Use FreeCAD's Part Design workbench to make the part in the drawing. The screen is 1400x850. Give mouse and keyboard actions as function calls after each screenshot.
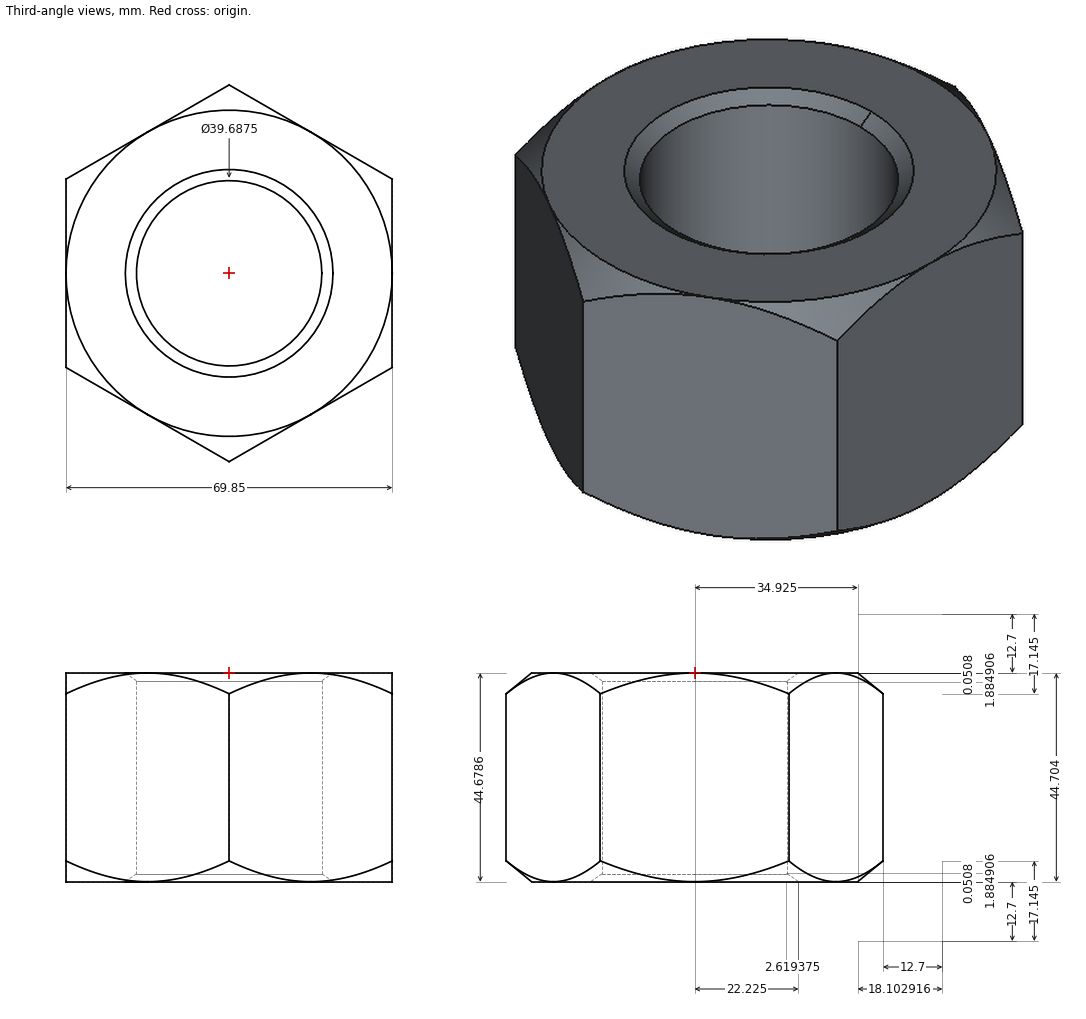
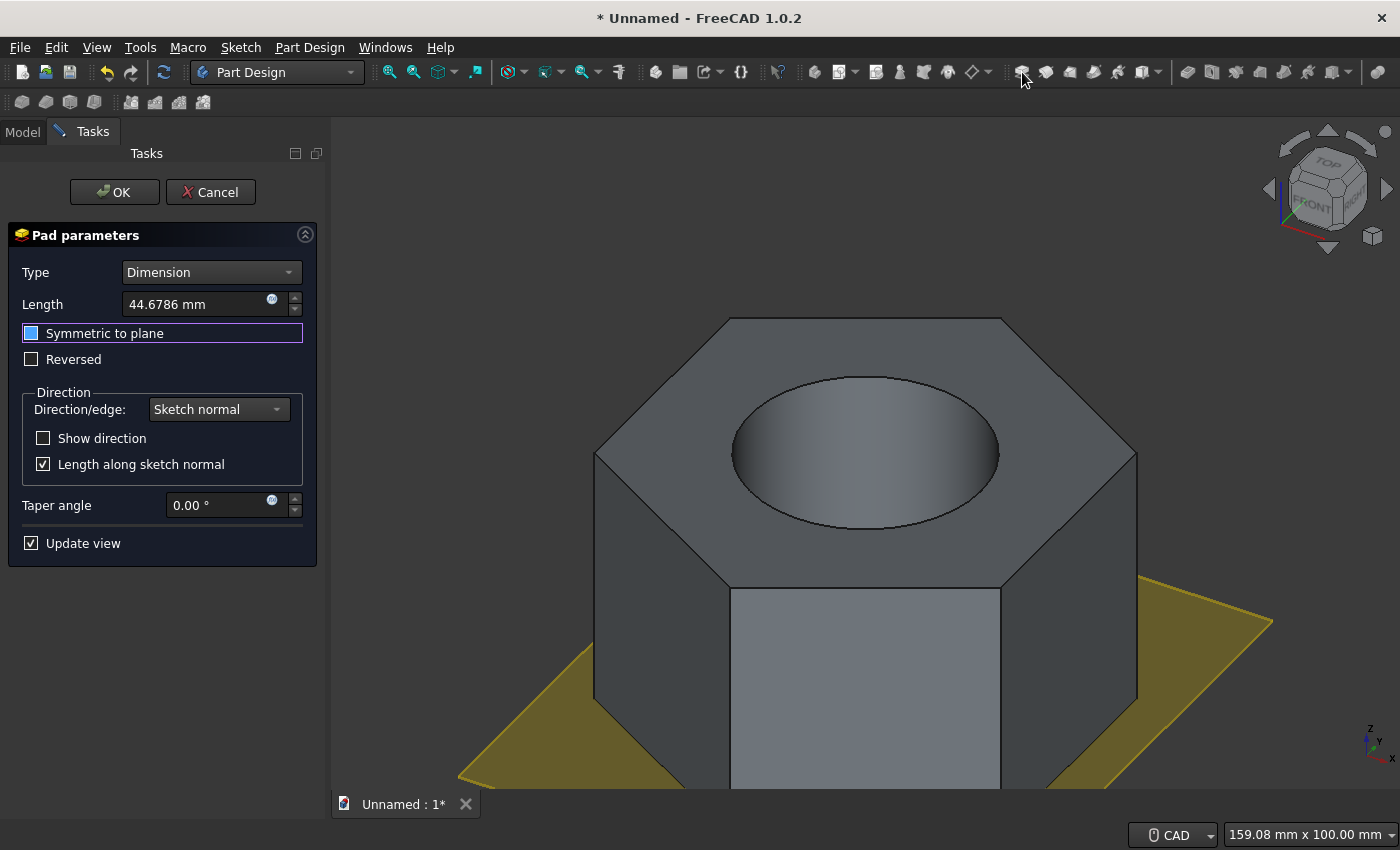
click(115, 192)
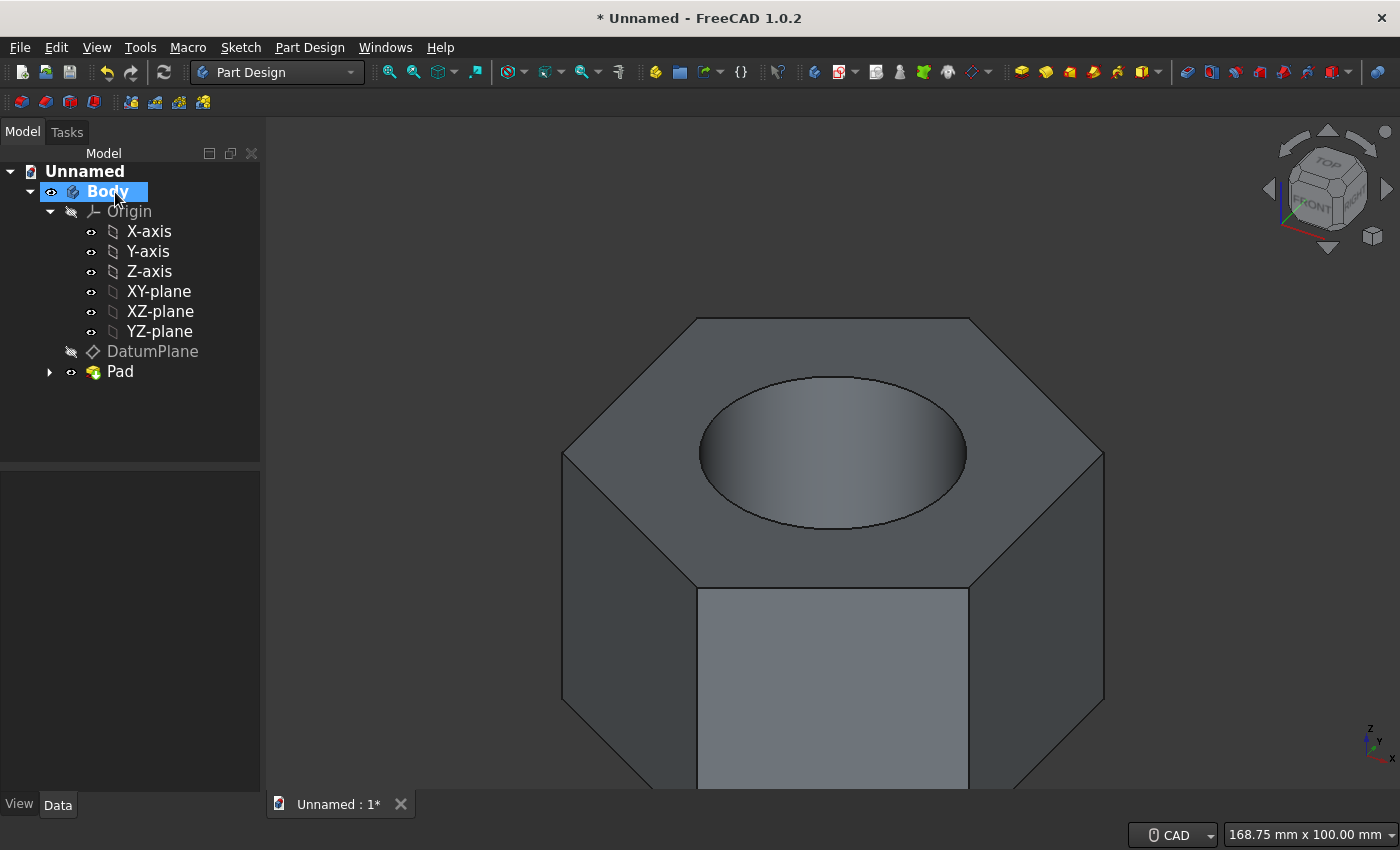
click(390, 72)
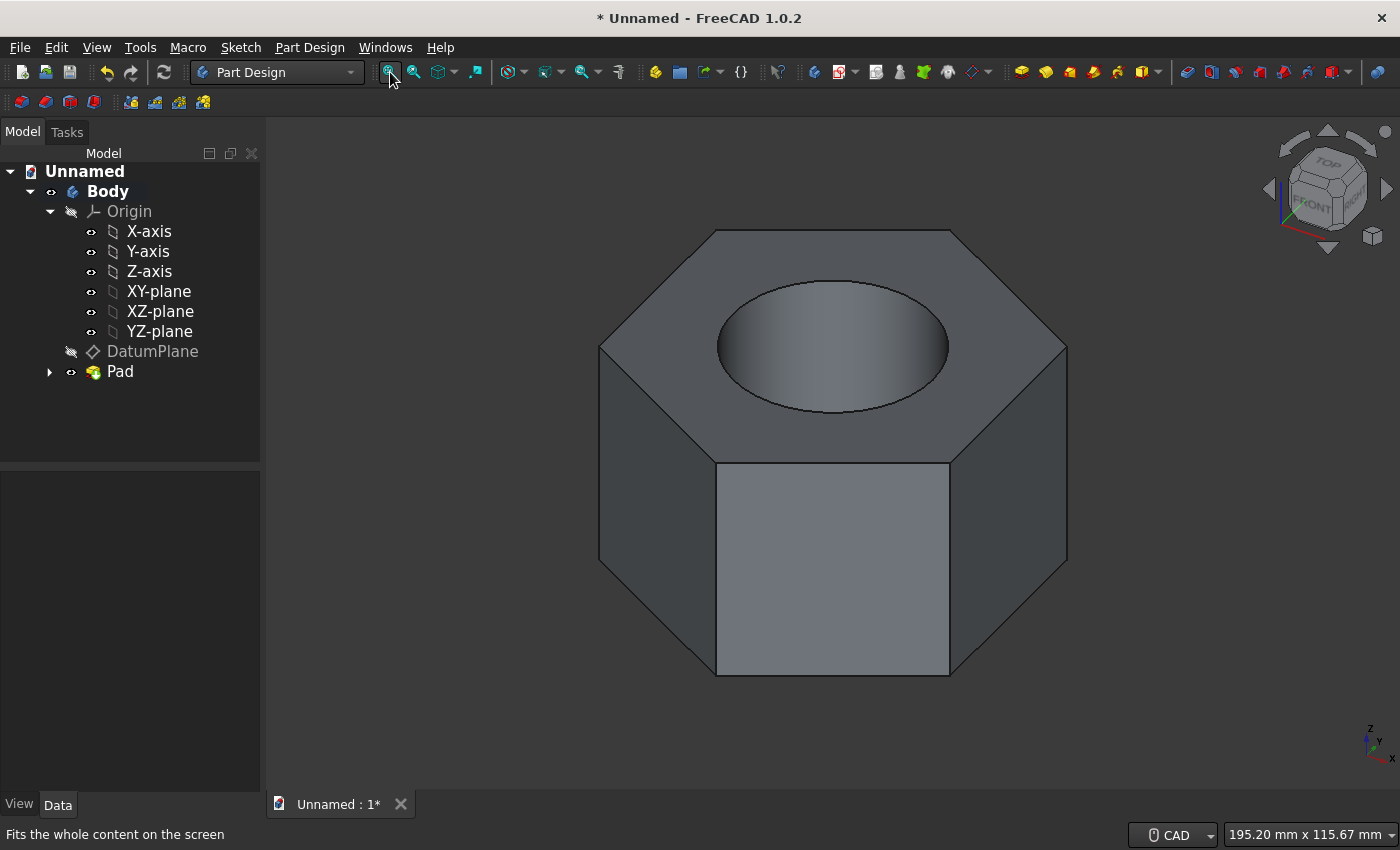
click(840, 72)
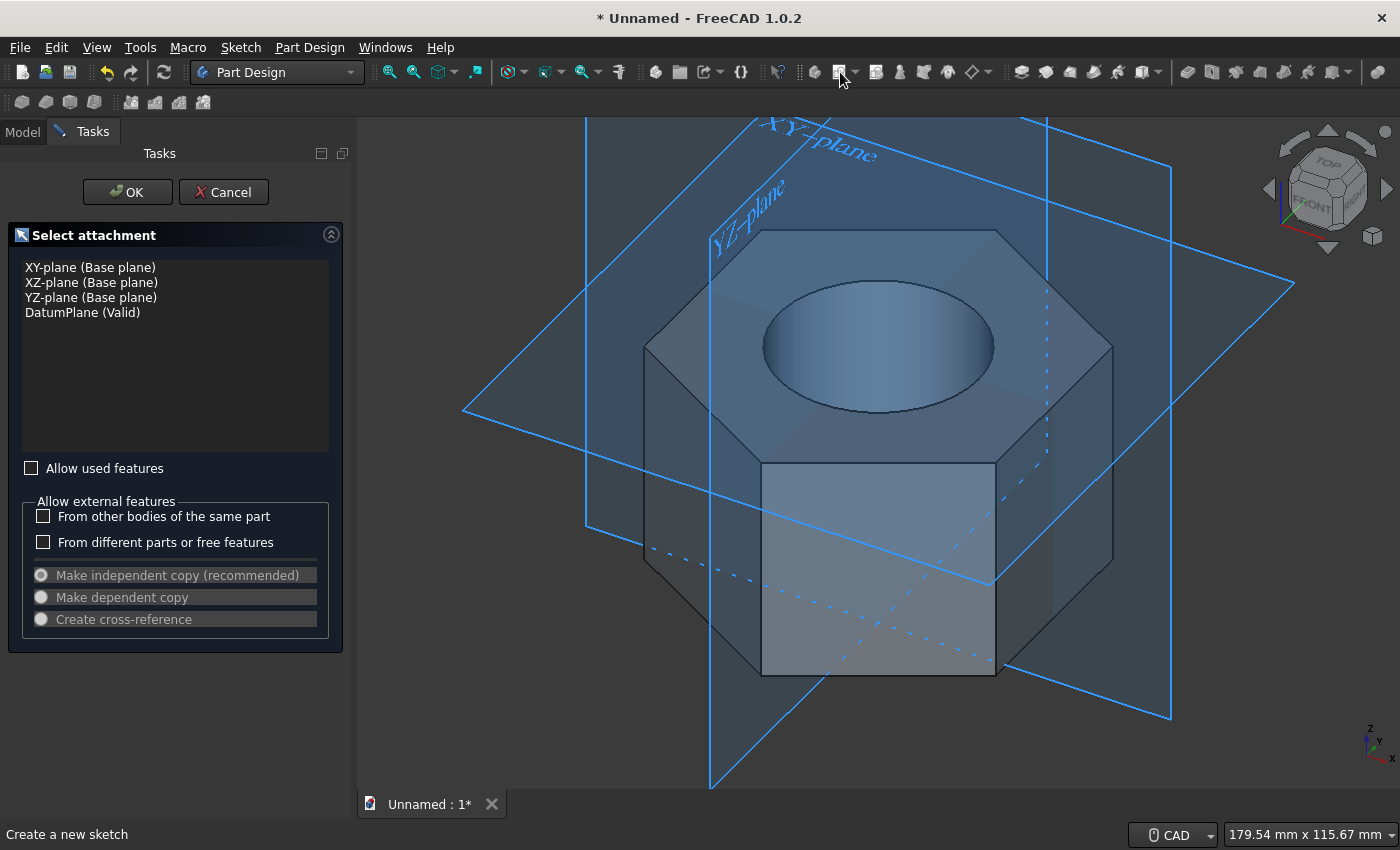
click(82, 298)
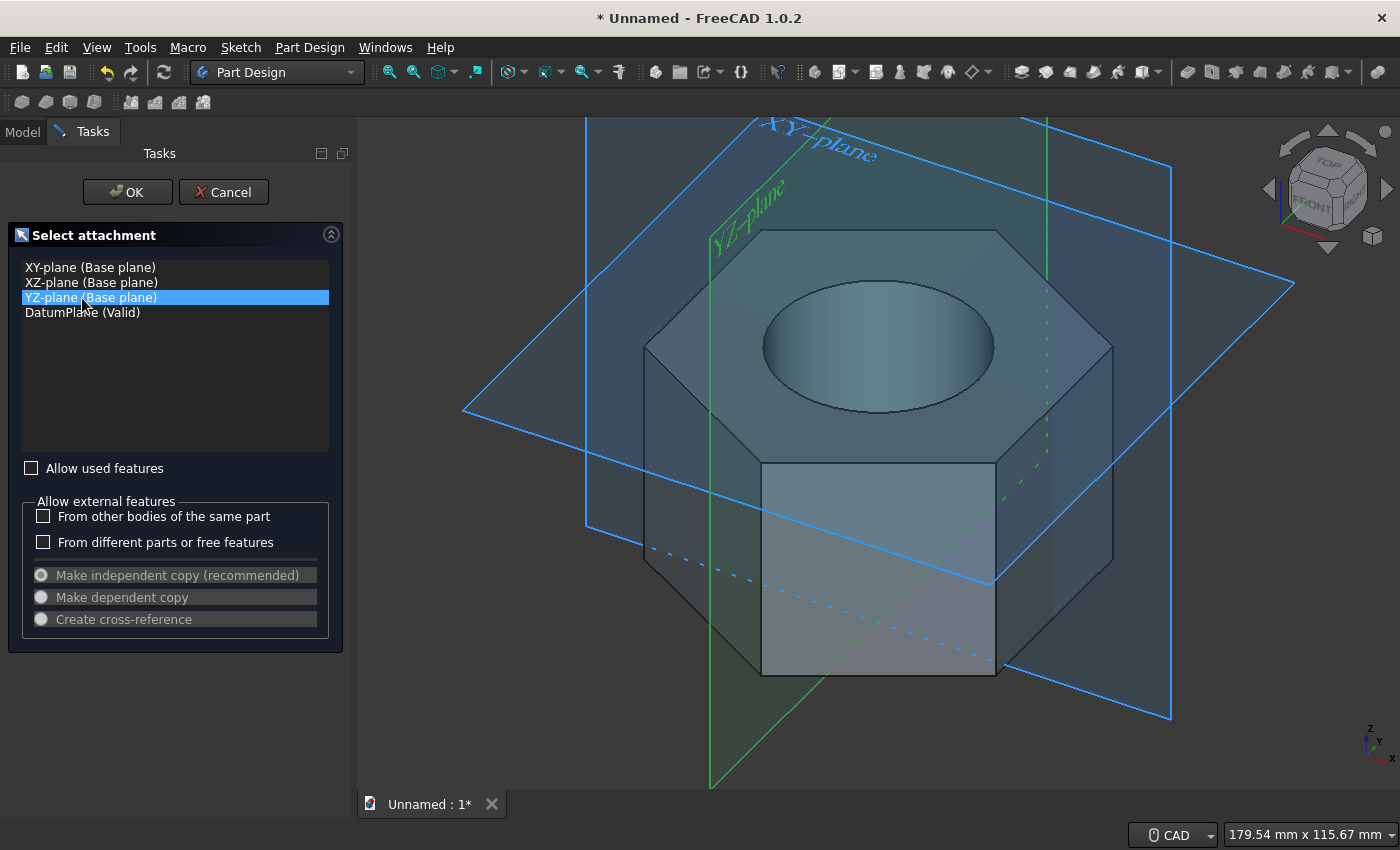
click(128, 192)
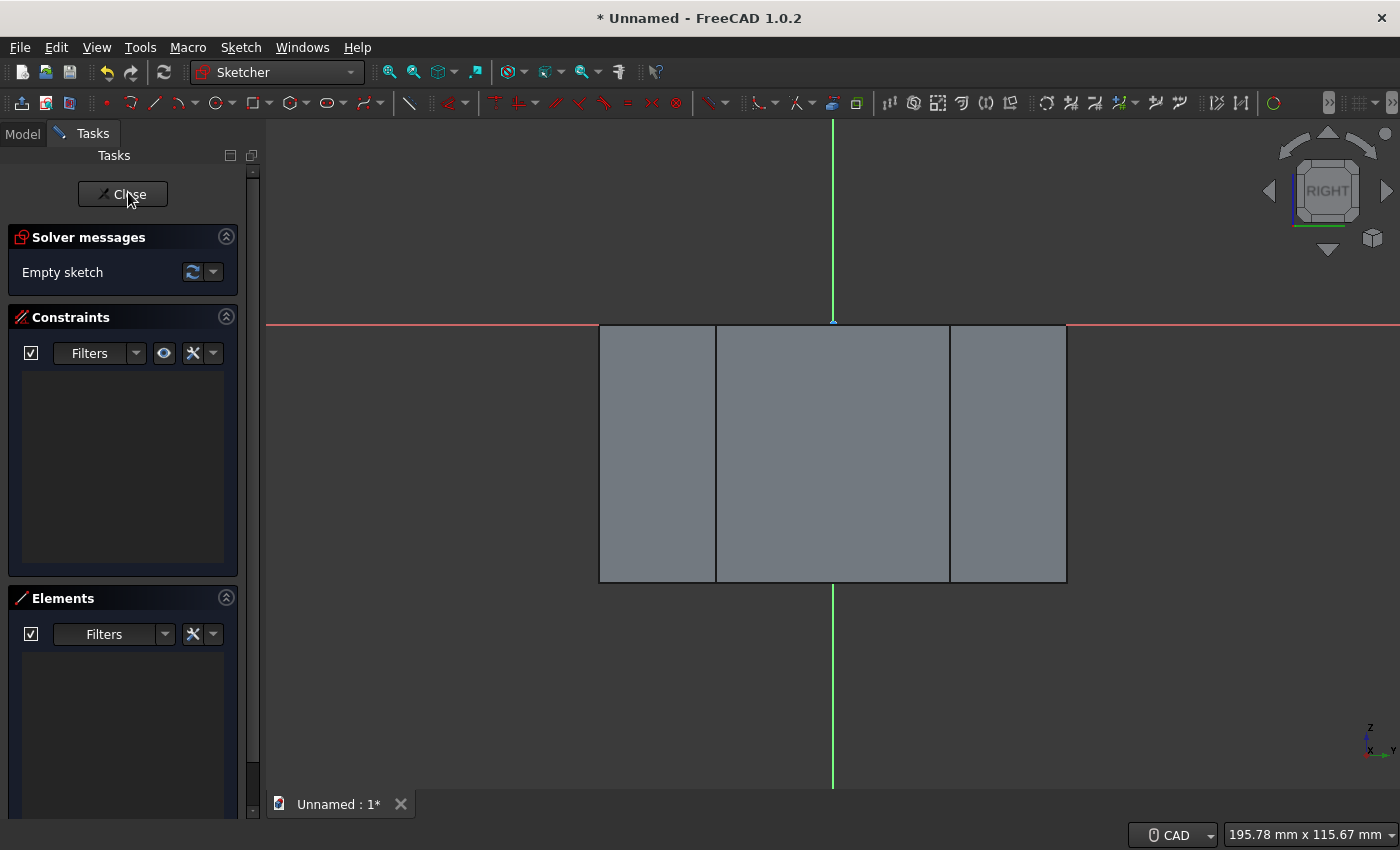
key(q)
key(s)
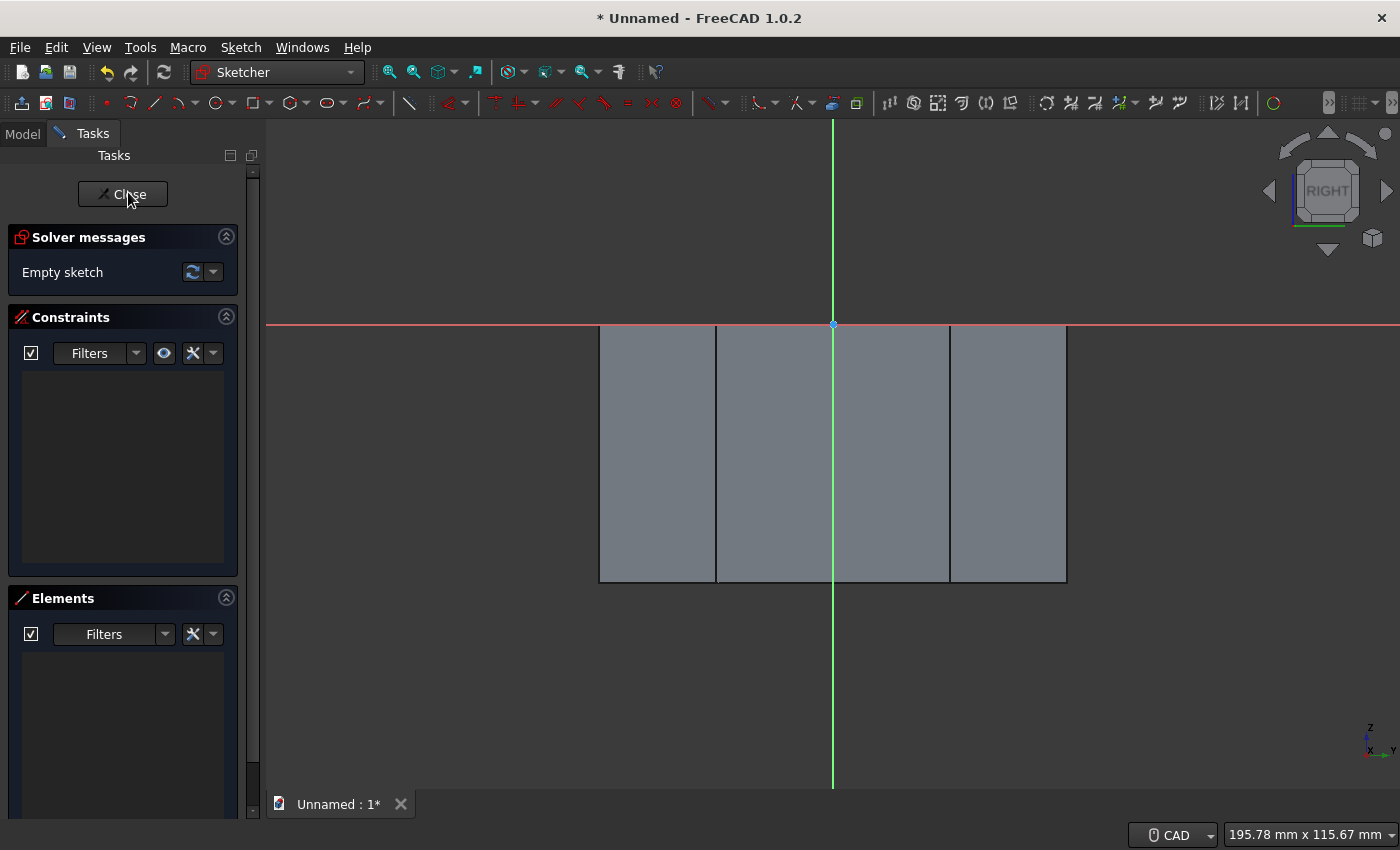
click(132, 104)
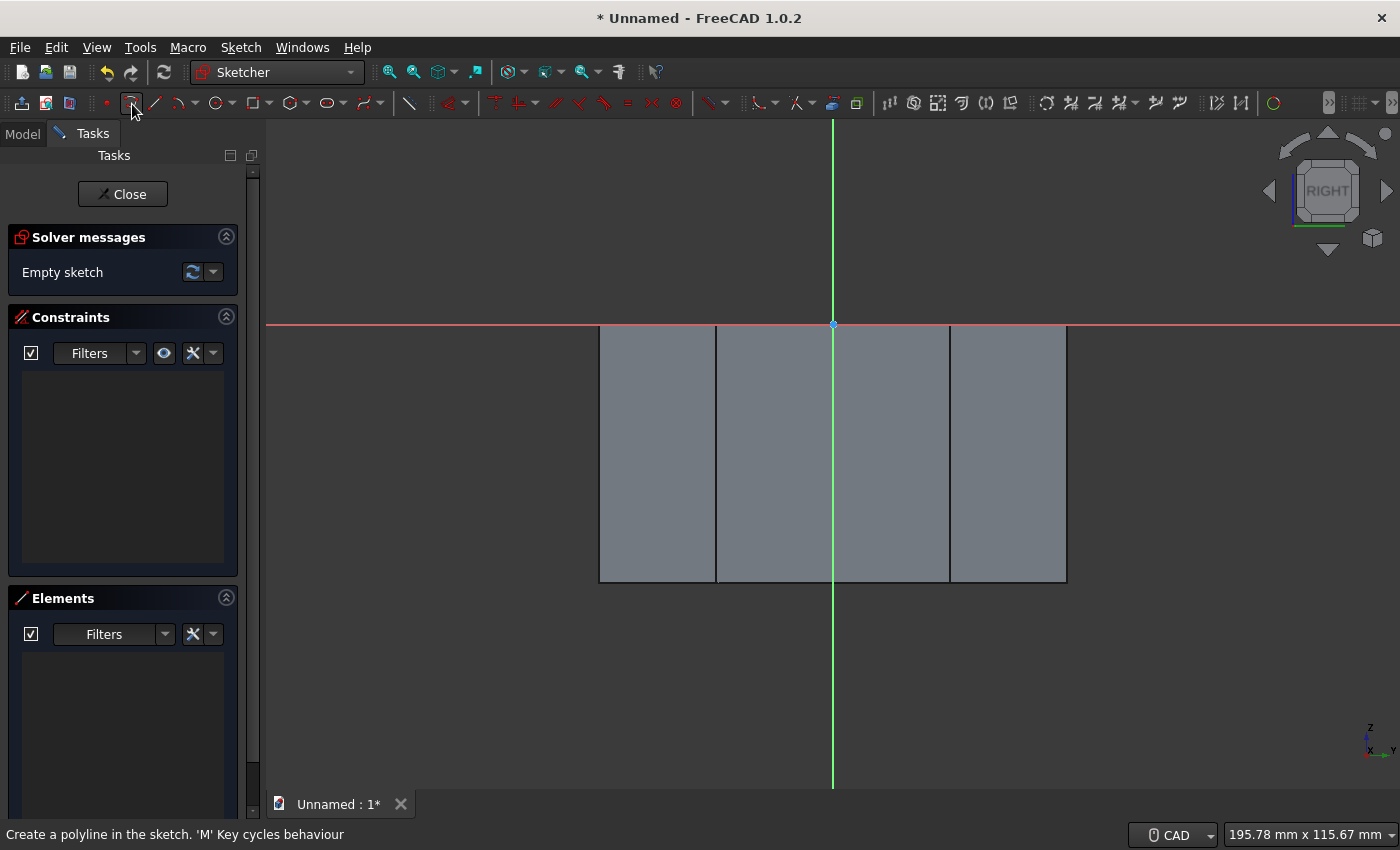
click(1035, 583)
click(1035, 657)
click(1140, 657)
click(1140, 558)
click(1067, 558)
click(1035, 584)